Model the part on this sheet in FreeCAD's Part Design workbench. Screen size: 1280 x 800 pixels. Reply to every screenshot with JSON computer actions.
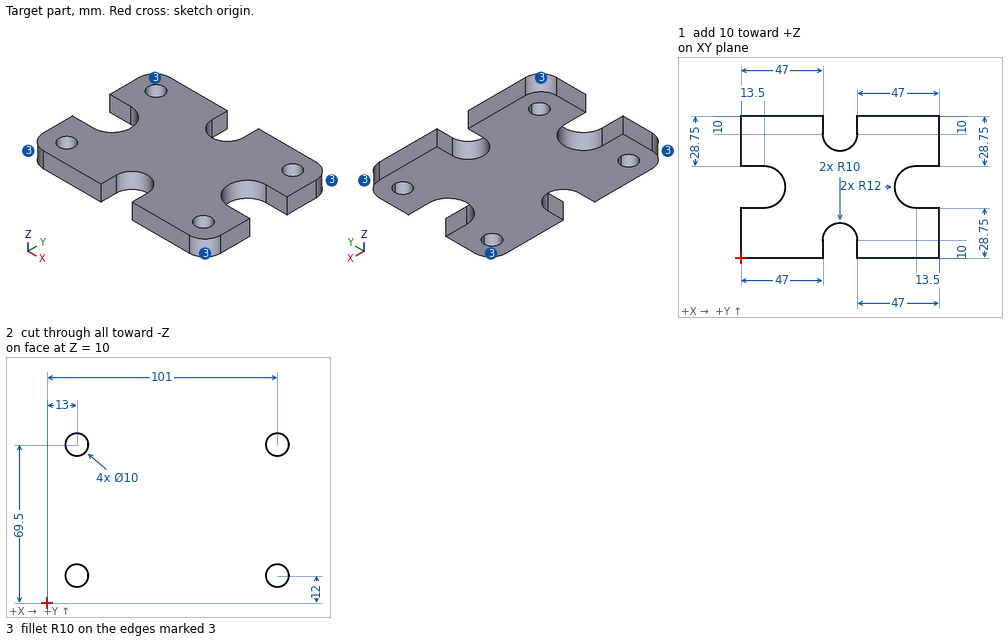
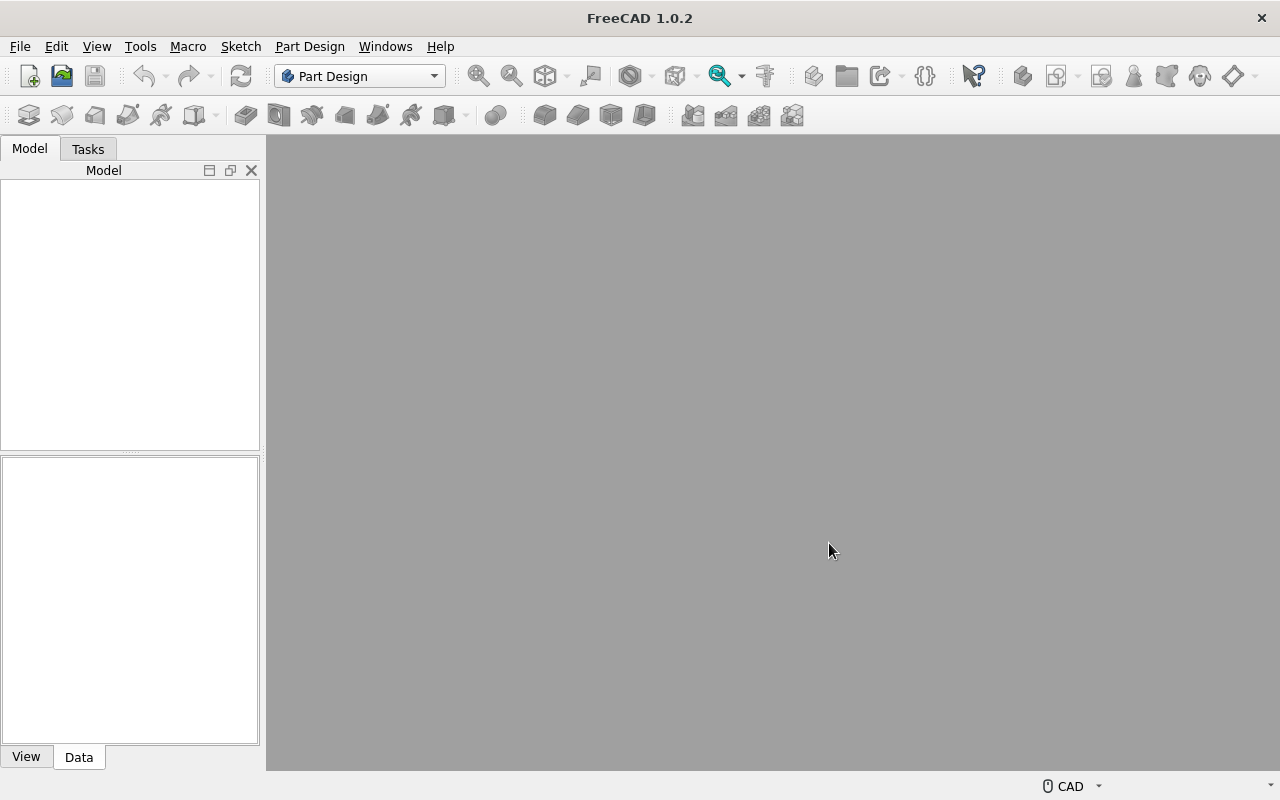
{"action": "left_click", "coordinate": [29, 76]}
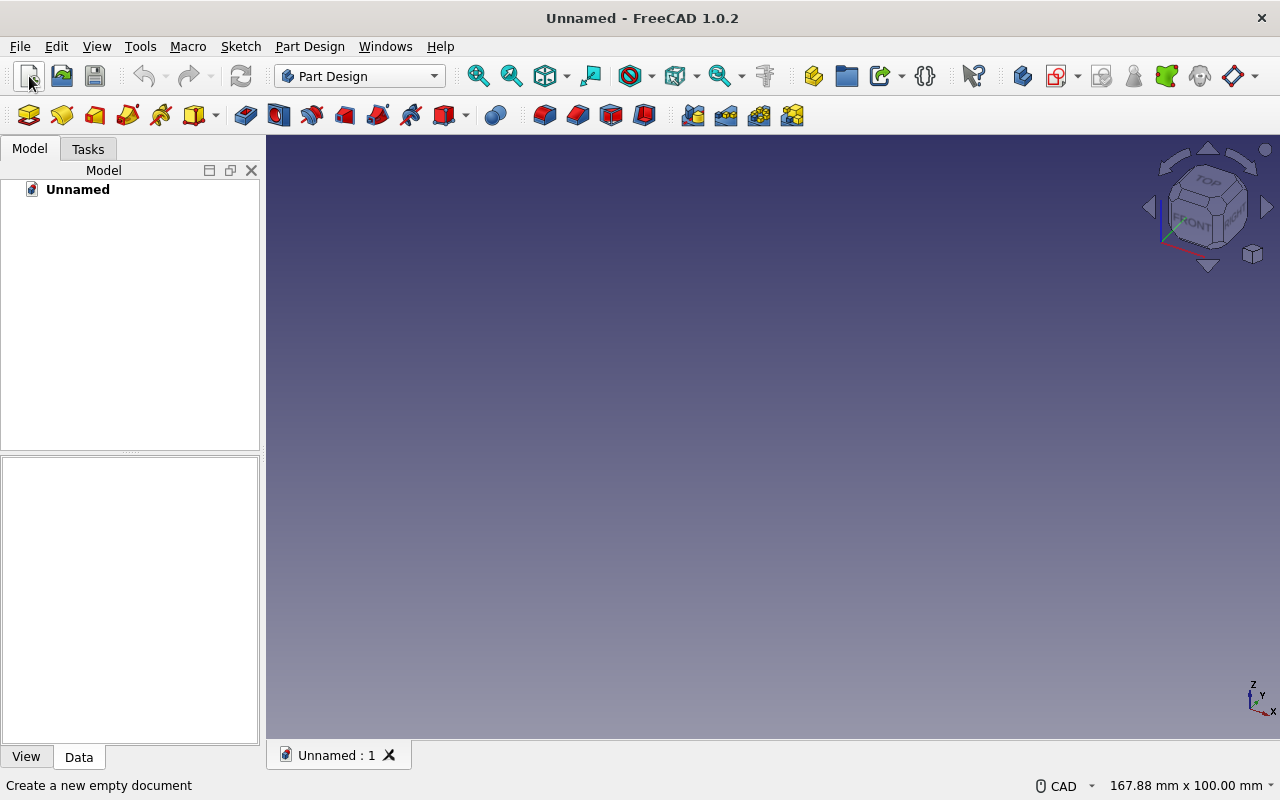
{"action": "left_click", "coordinate": [1056, 76]}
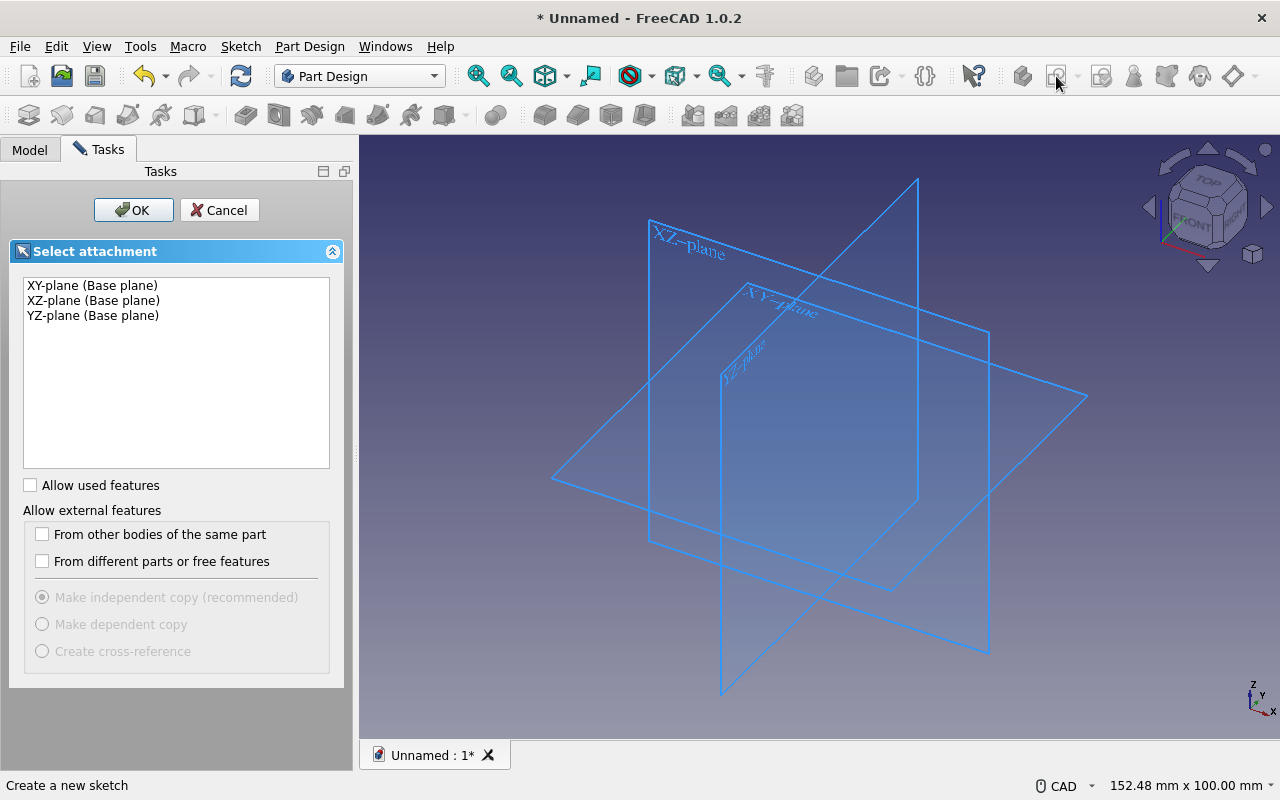
{"action": "left_click", "coordinate": [84, 286]}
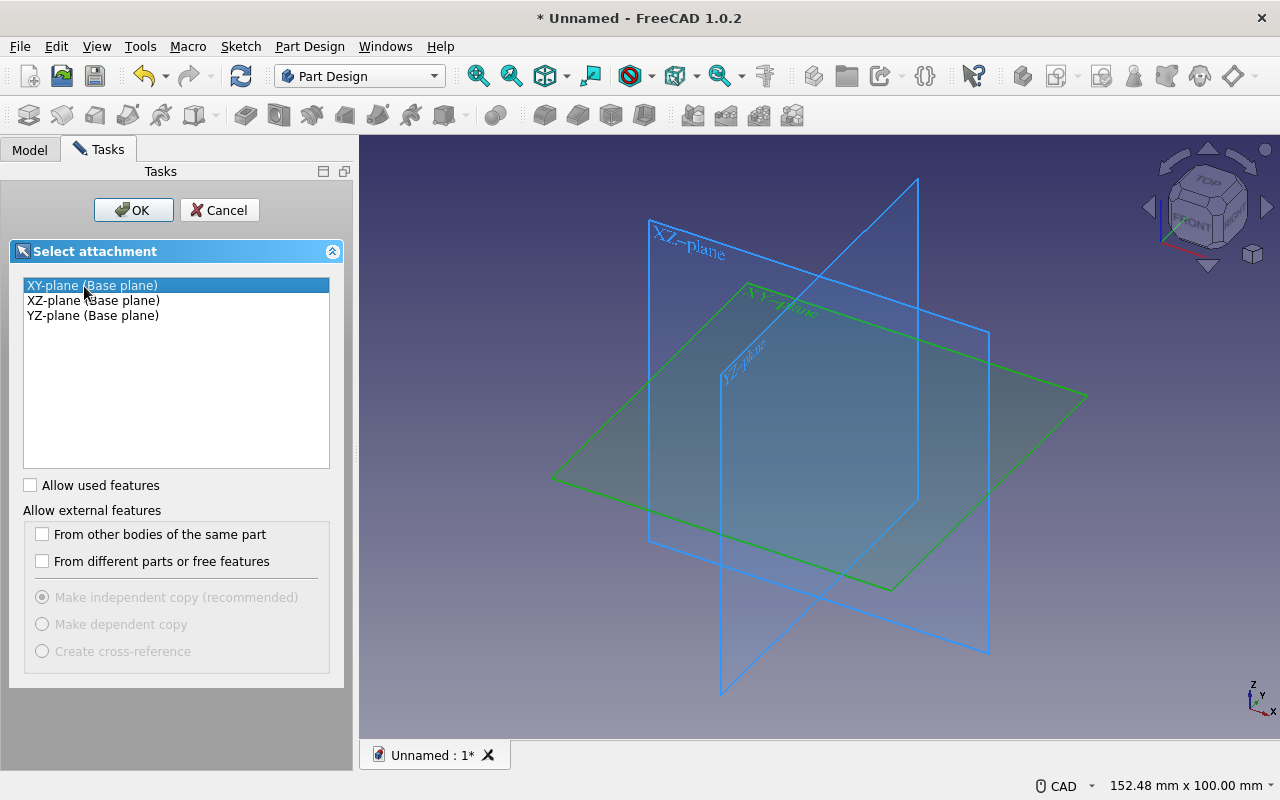
{"action": "left_click", "coordinate": [134, 210]}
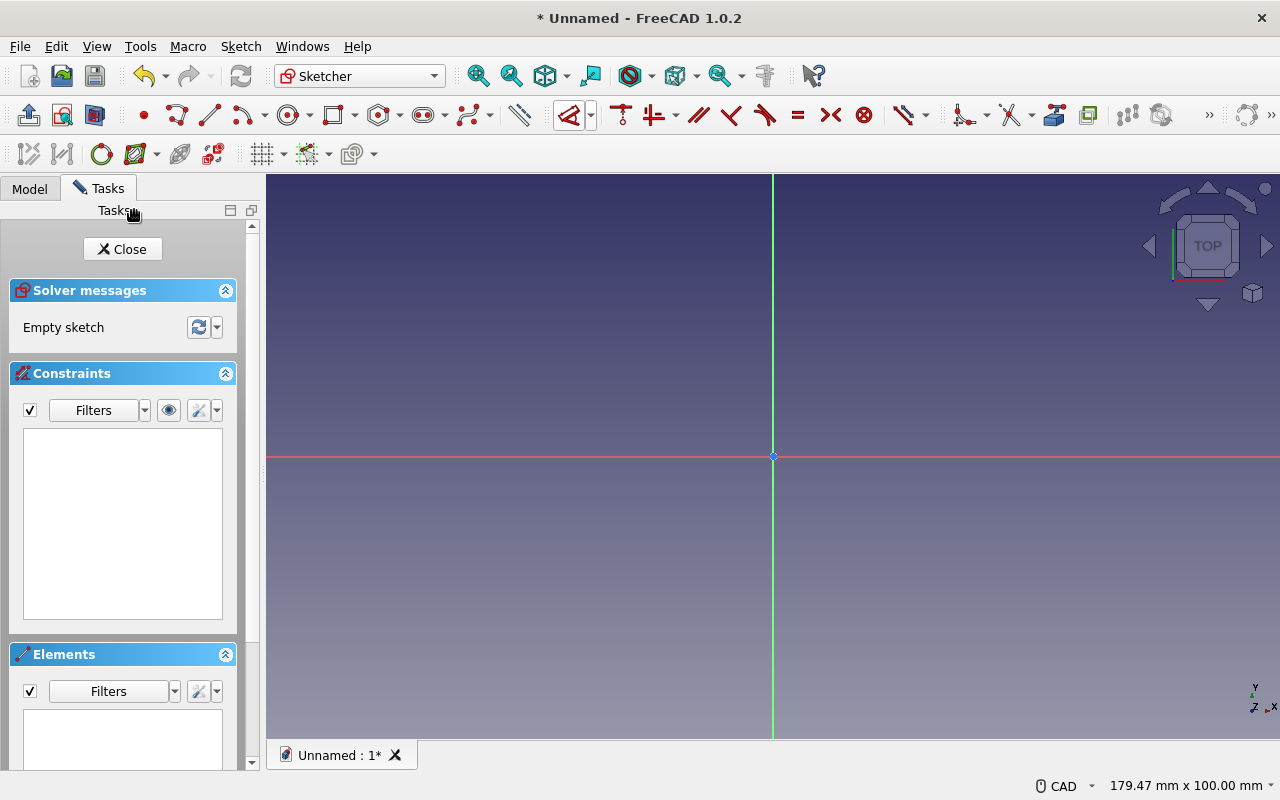
{"action": "scroll", "coordinate": [294, 711], "scroll_direction": "down", "scroll_amount": 2}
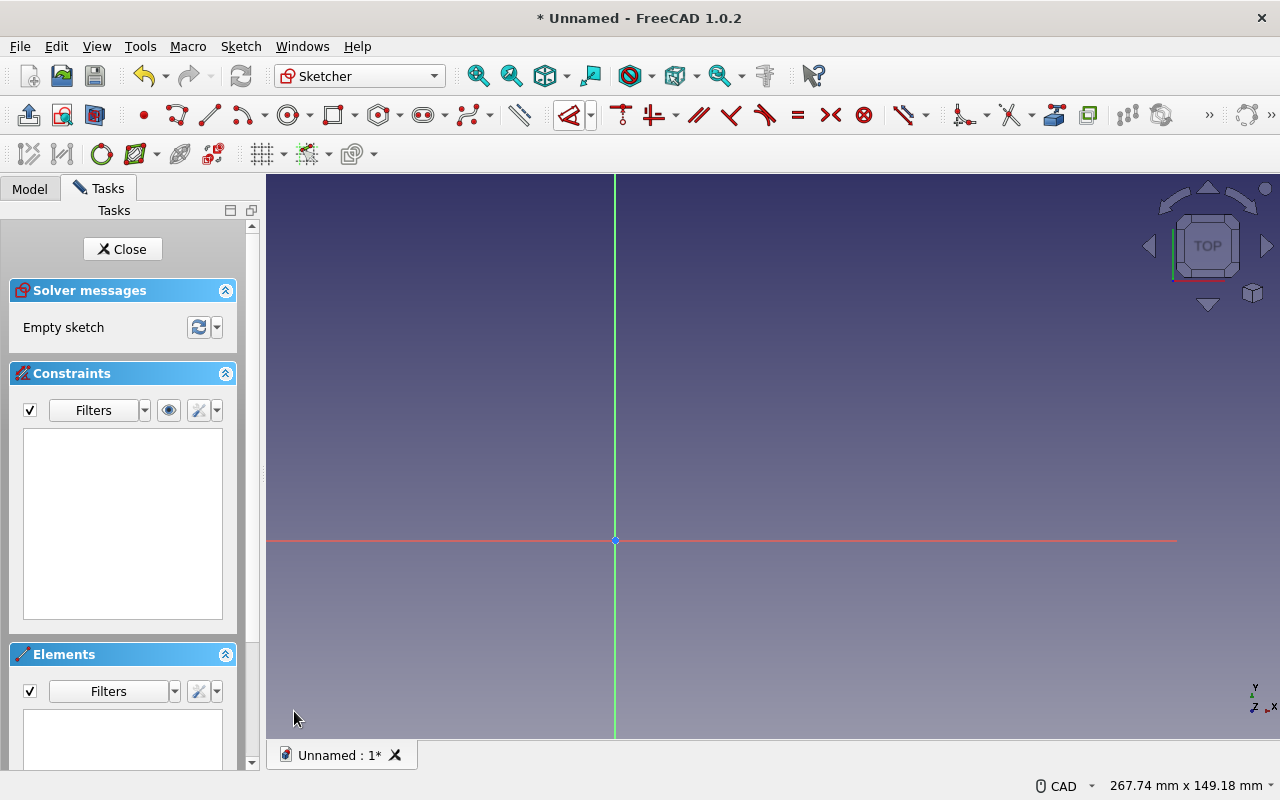
{"action": "left_click", "coordinate": [177, 116]}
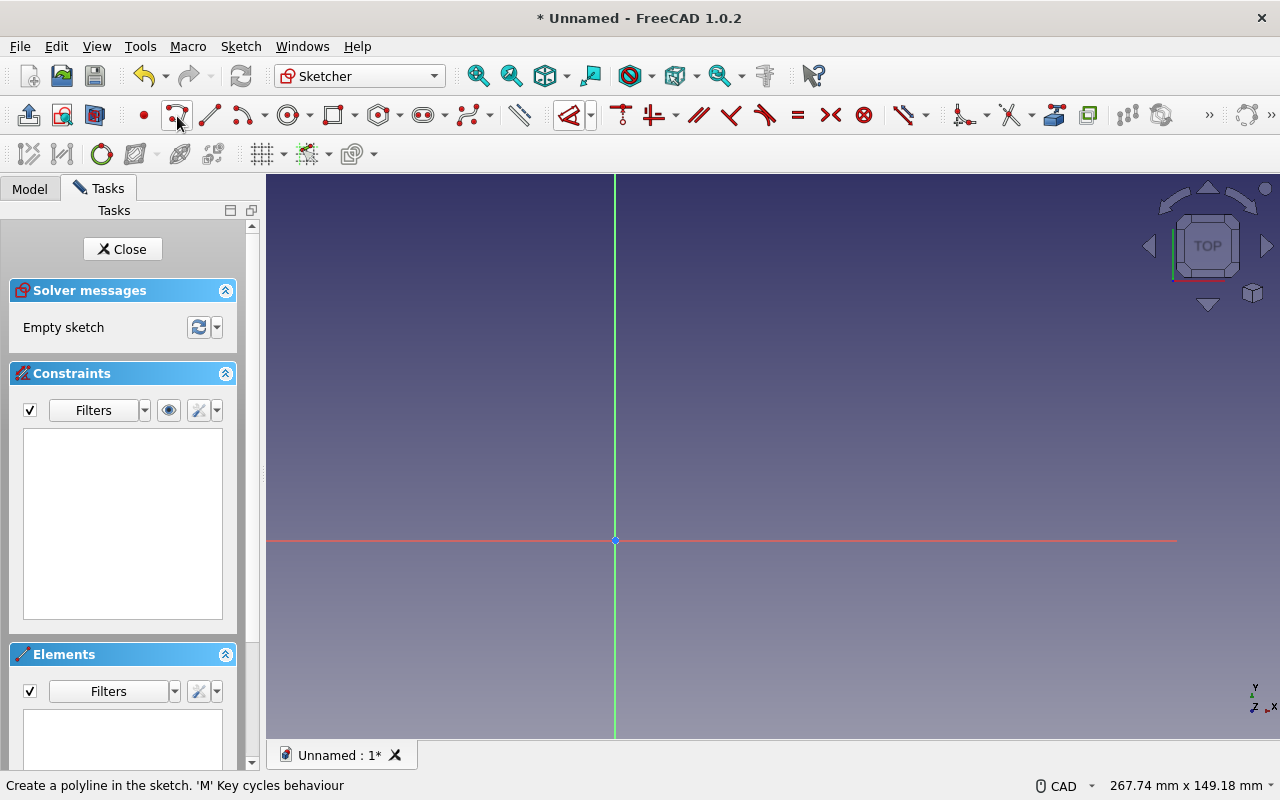
{"action": "left_click", "coordinate": [869, 503]}
{"action": "left_click", "coordinate": [869, 541]}
{"action": "left_click", "coordinate": [1047, 532]}
{"action": "left_click", "coordinate": [1047, 432]}
{"action": "left_click", "coordinate": [996, 432]}
{"action": "right_click", "coordinate": [996, 432]}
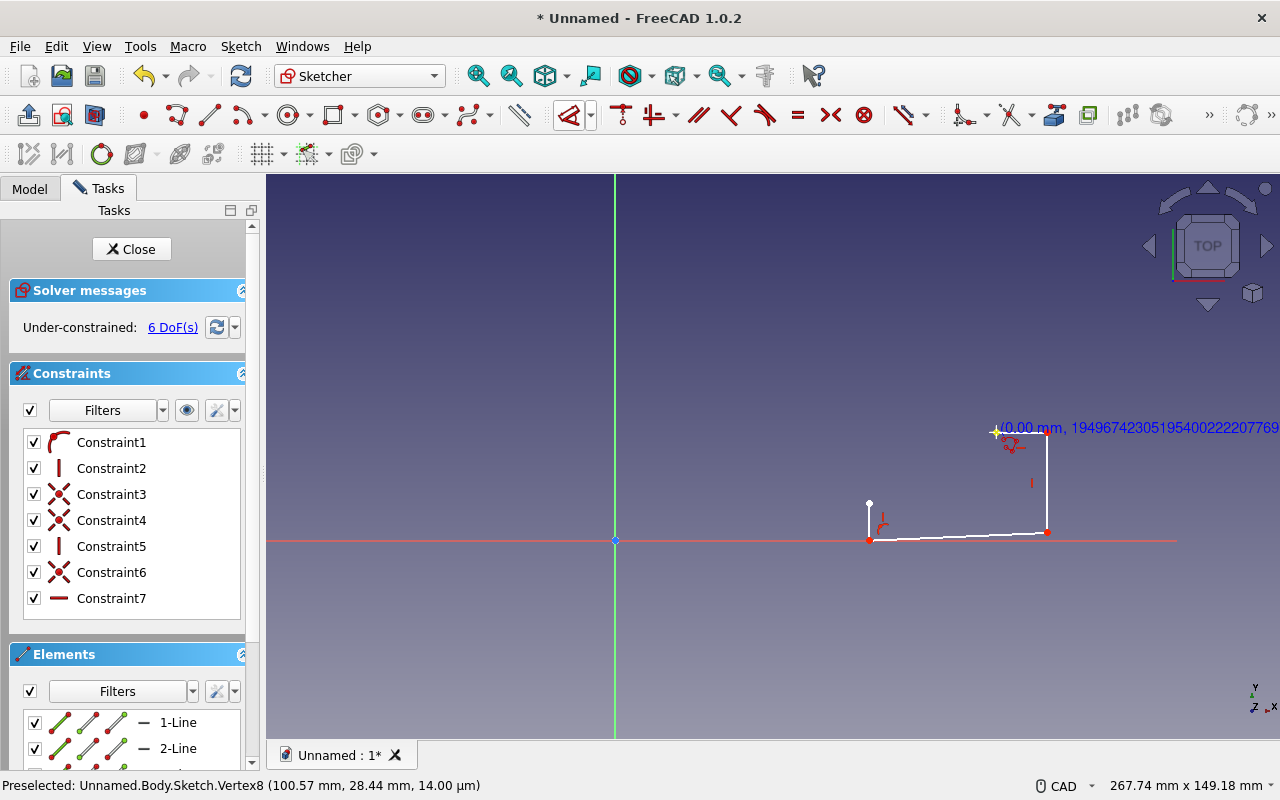
{"action": "left_click", "coordinate": [996, 341]}
{"action": "left_click", "coordinate": [1047, 341]}
{"action": "left_click", "coordinate": [1047, 232]}
{"action": "left_click", "coordinate": [869, 232]}
{"action": "left_click", "coordinate": [869, 270]}
{"action": "right_click", "coordinate": [869, 270]}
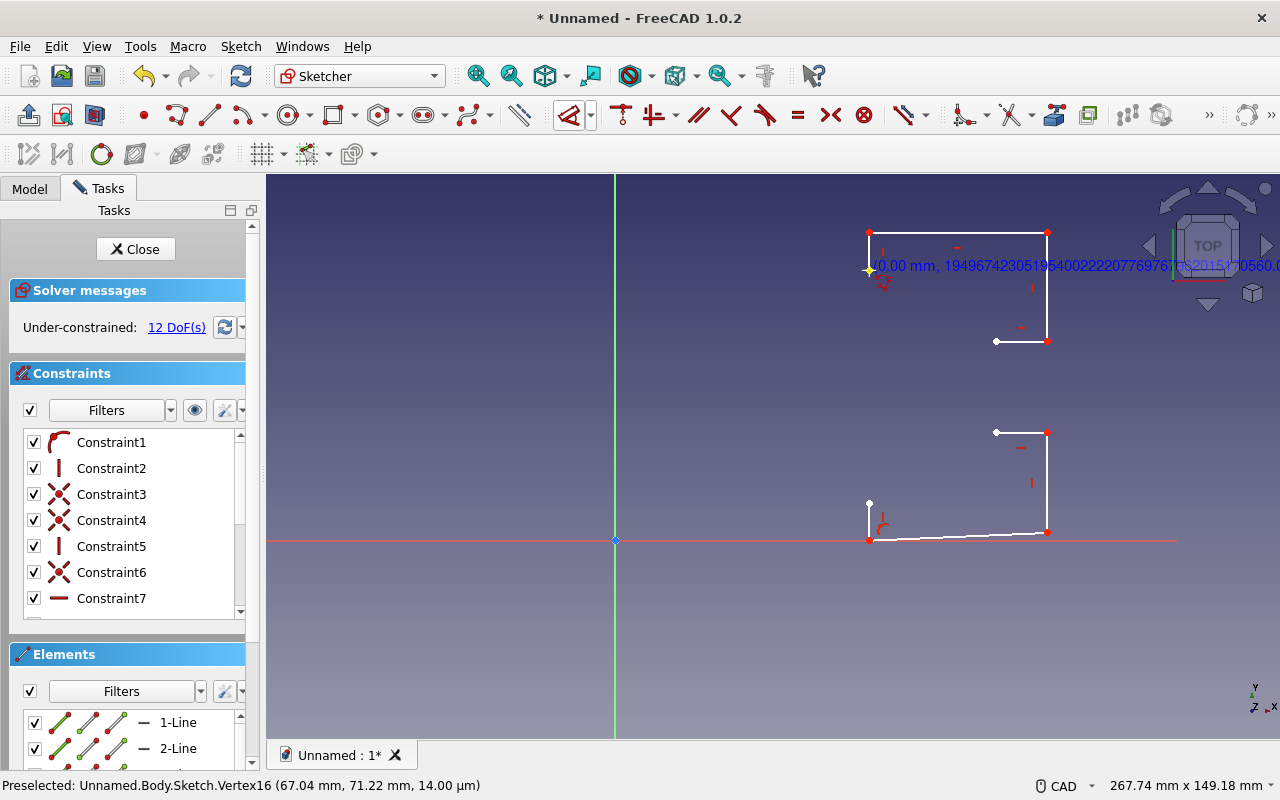
{"action": "left_click", "coordinate": [793, 270]}
{"action": "left_click", "coordinate": [793, 232]}
{"action": "left_click", "coordinate": [615, 232]}
{"action": "left_click", "coordinate": [624, 341]}
{"action": "left_click", "coordinate": [666, 341]}
{"action": "right_click", "coordinate": [666, 341]}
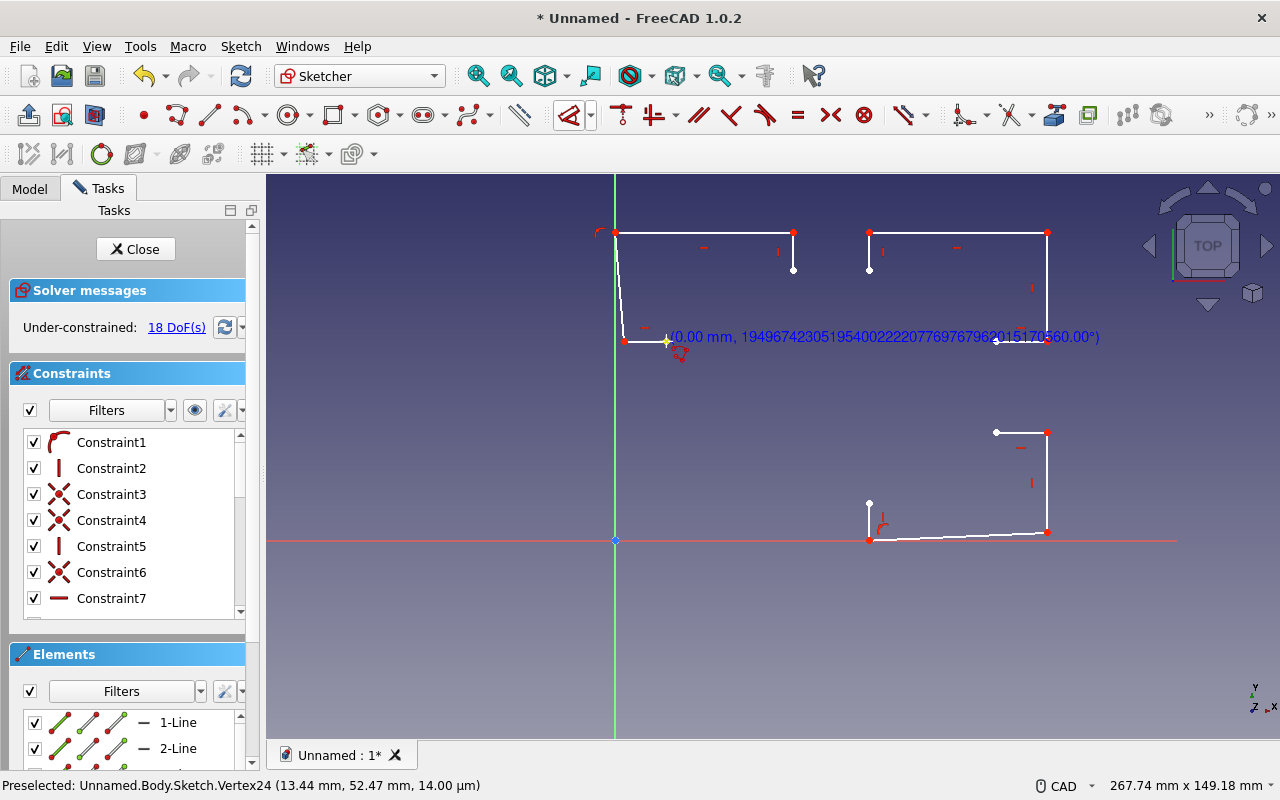
{"action": "left_click", "coordinate": [666, 432]}
{"action": "left_click", "coordinate": [615, 432]}
{"action": "left_click", "coordinate": [615, 541]}
{"action": "left_click", "coordinate": [793, 532]}
{"action": "left_click", "coordinate": [793, 503]}
{"action": "right_click", "coordinate": [793, 503]}